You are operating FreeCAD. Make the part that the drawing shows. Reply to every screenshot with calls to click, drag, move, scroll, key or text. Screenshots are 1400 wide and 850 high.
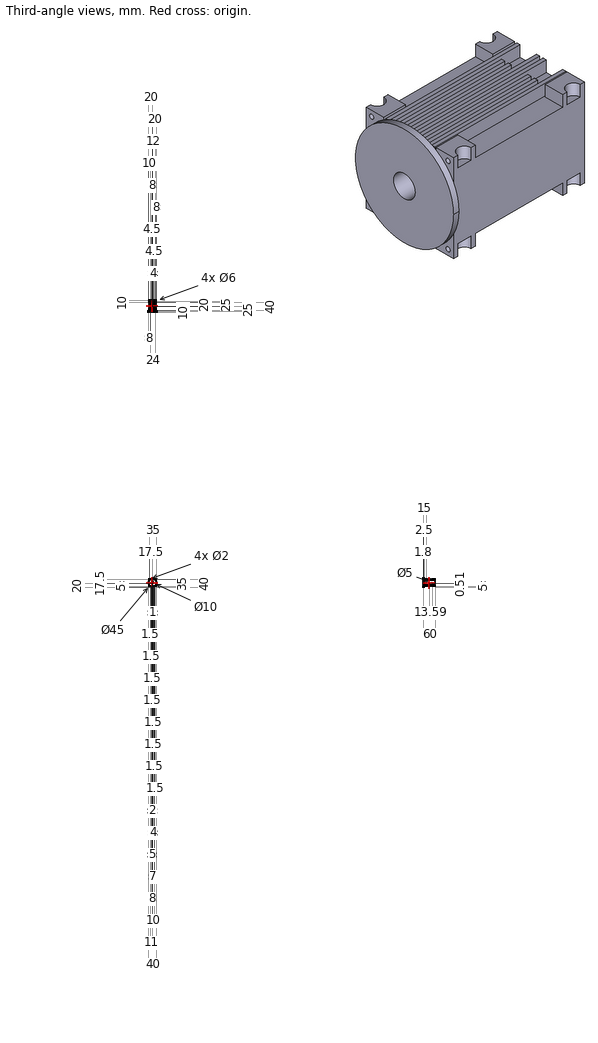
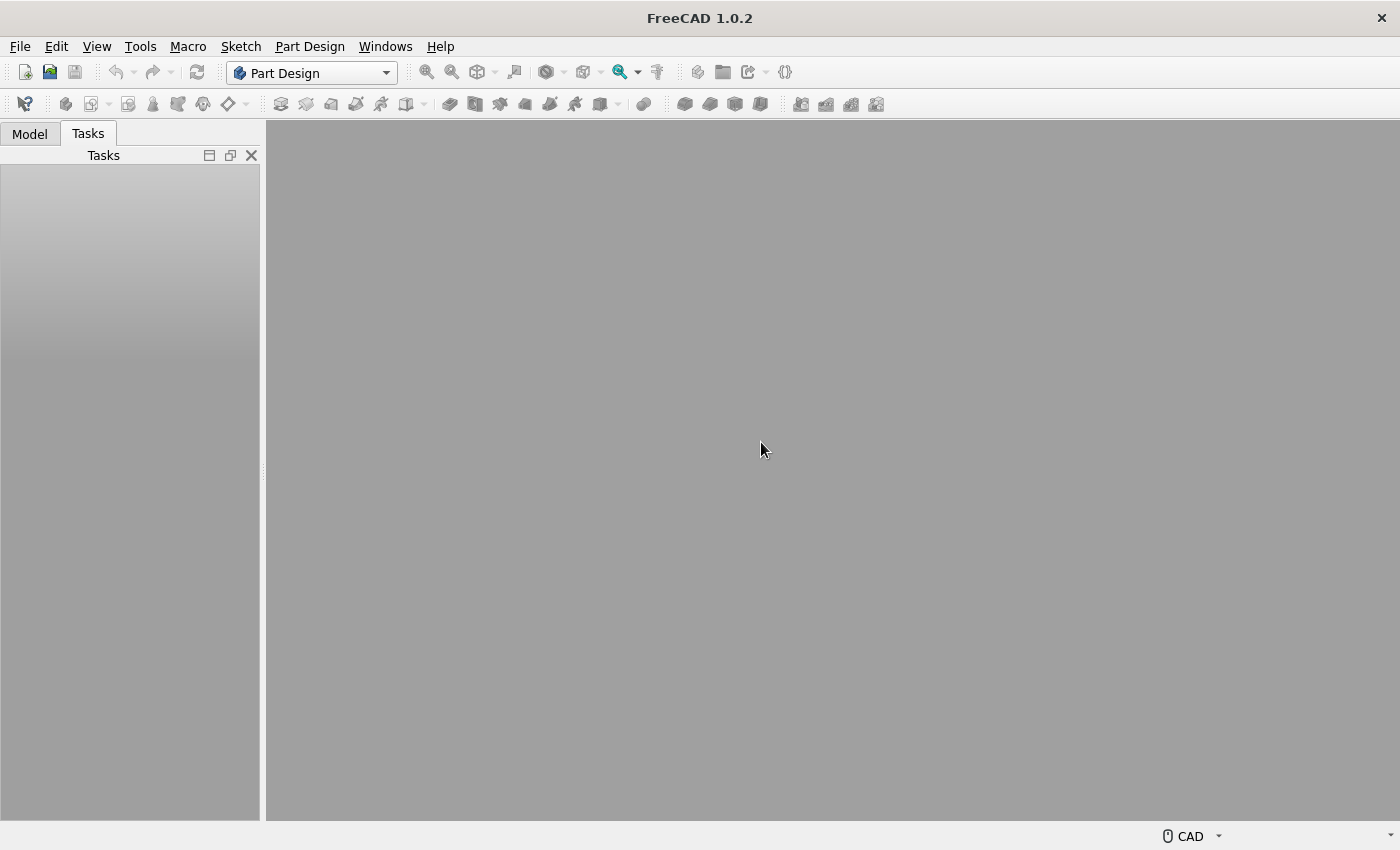
key(ctrl+n)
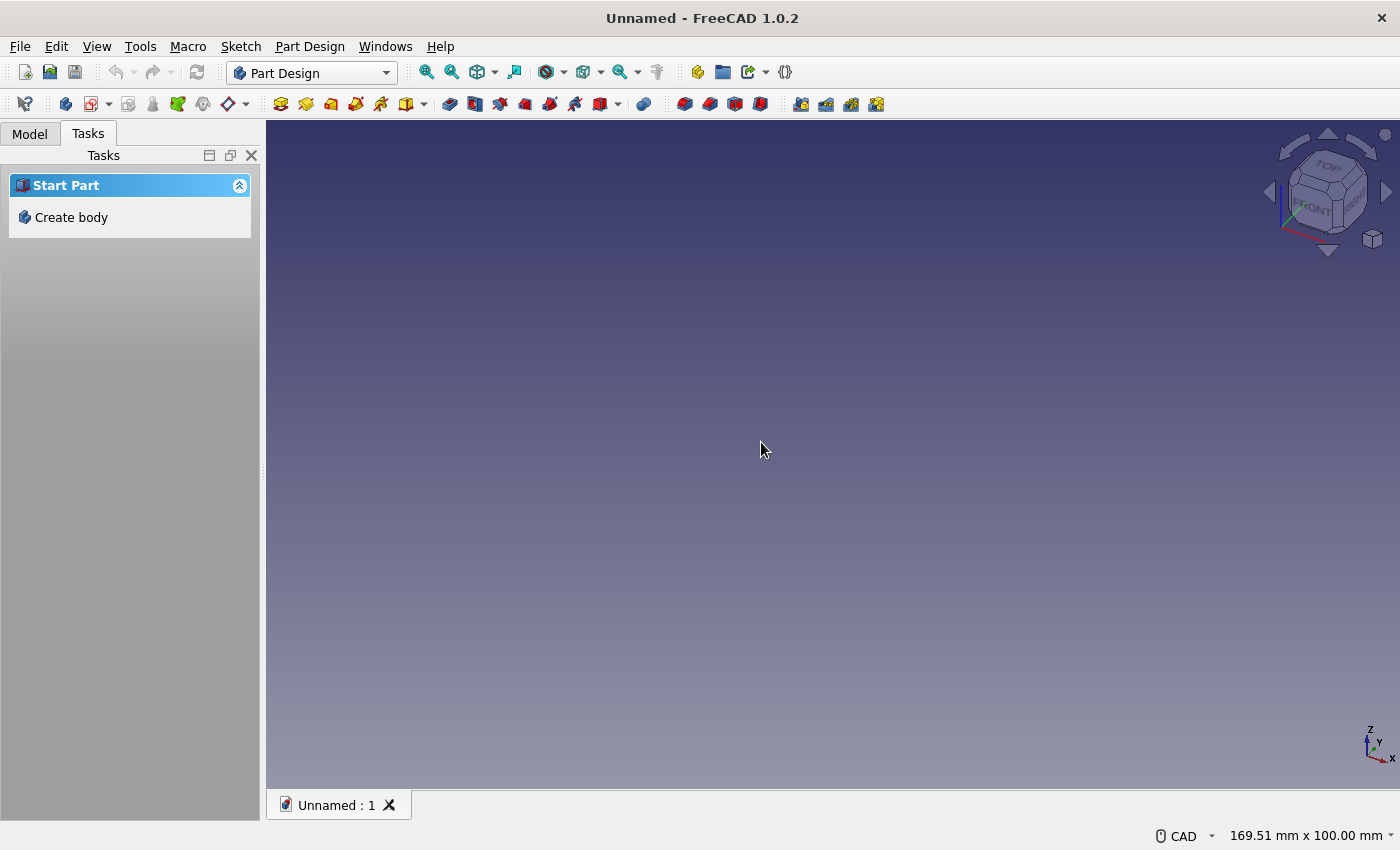
click(90, 104)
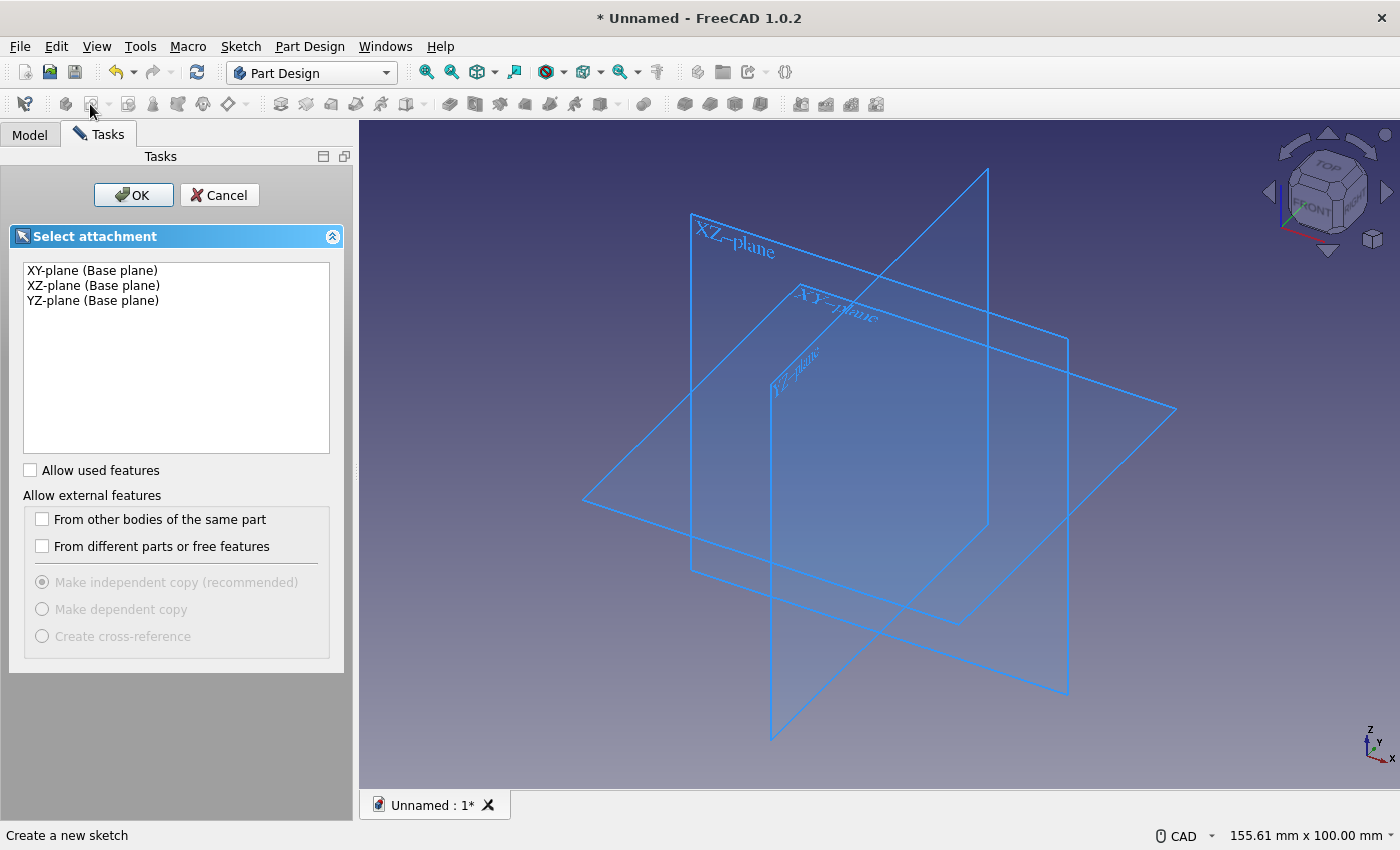
click(84, 286)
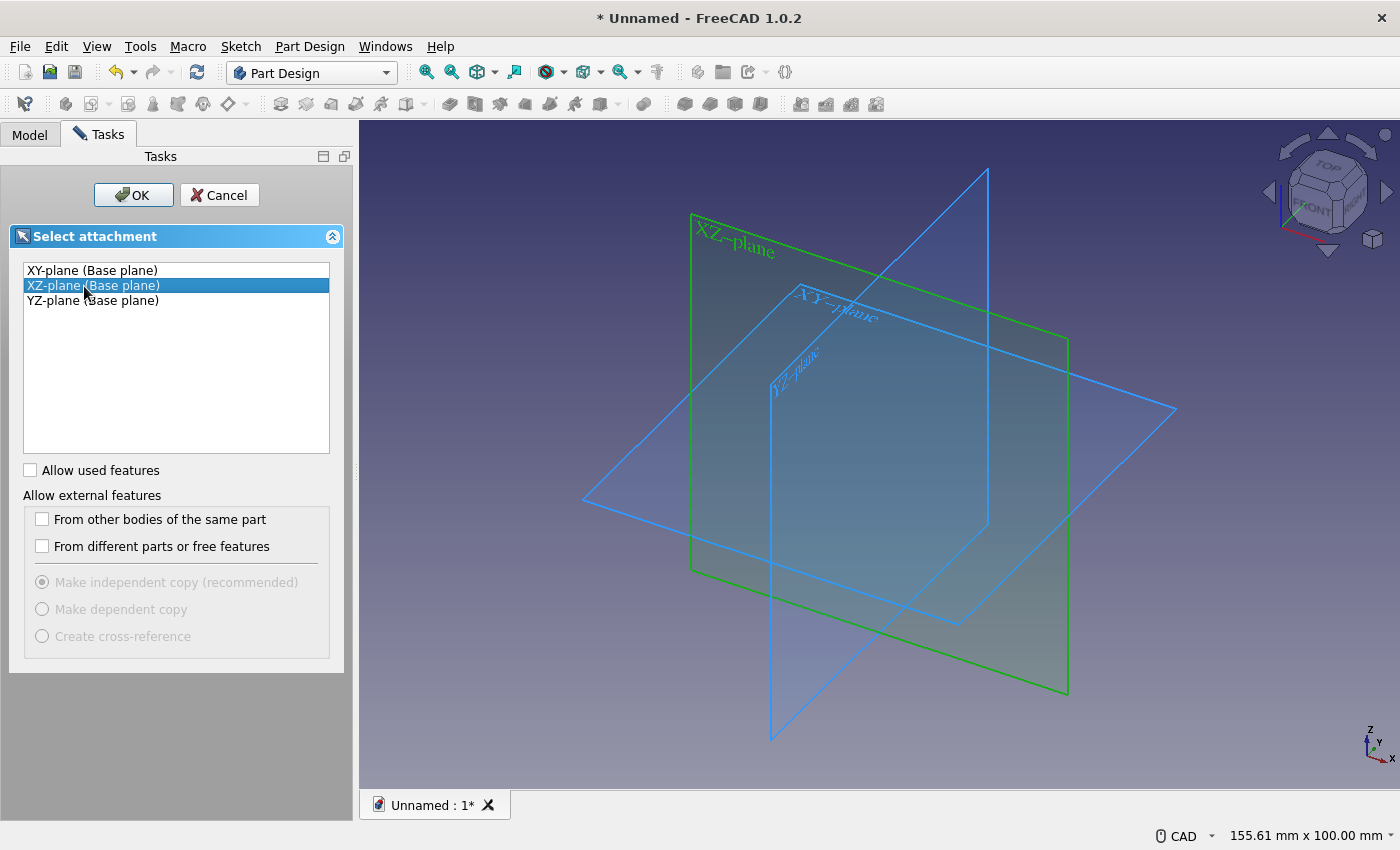
click(134, 195)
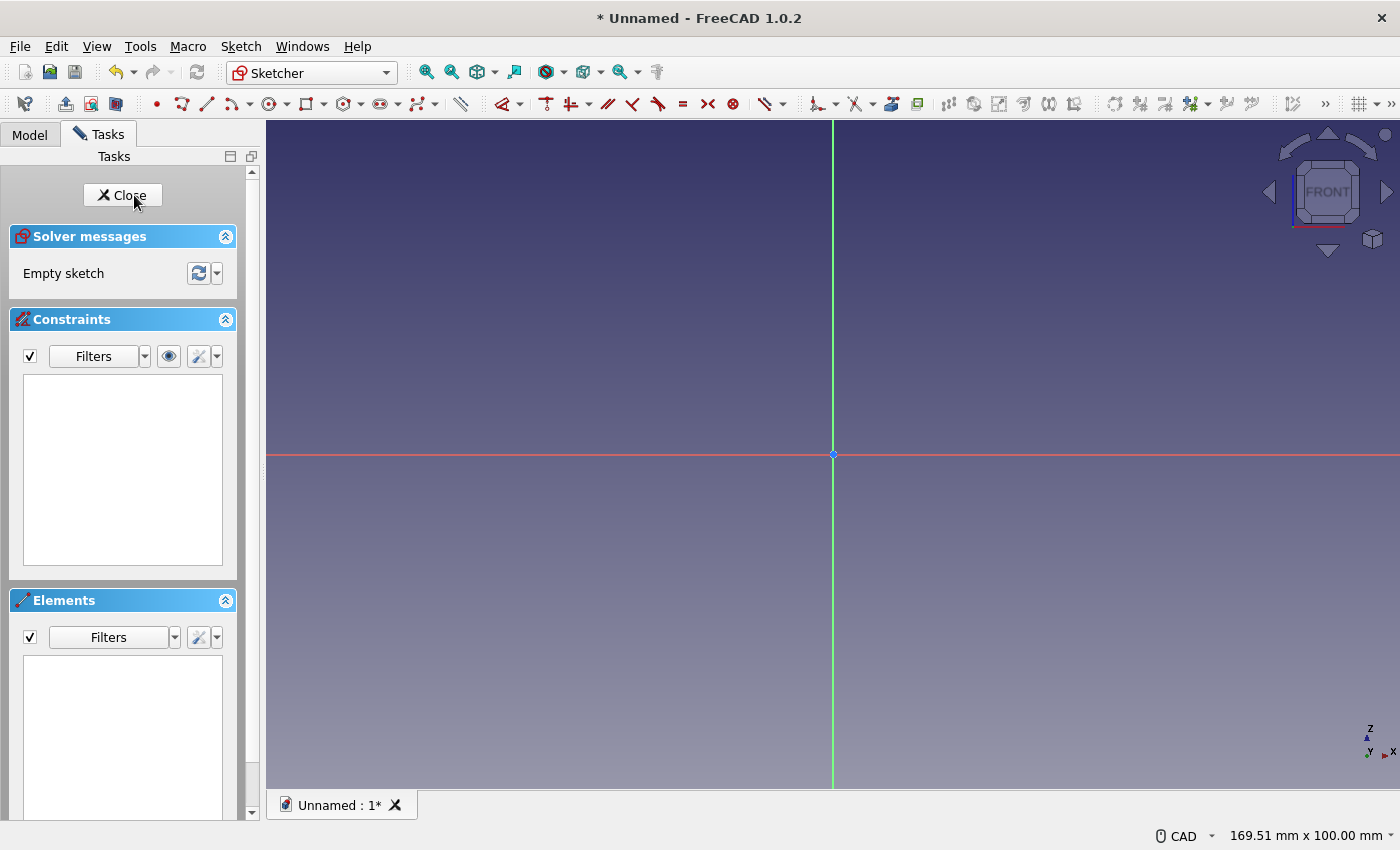
scroll(972, 455, up, 2)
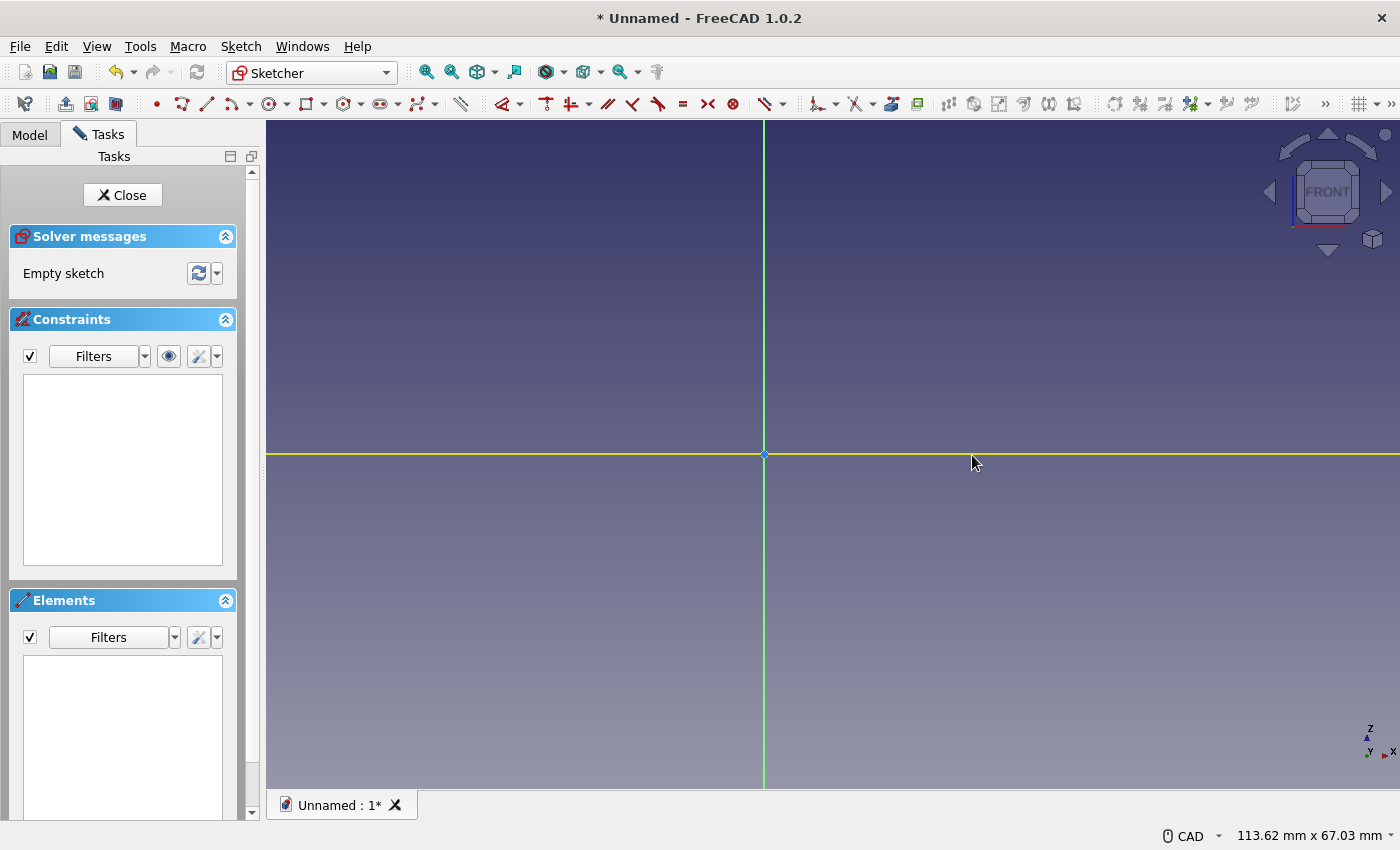
click(324, 104)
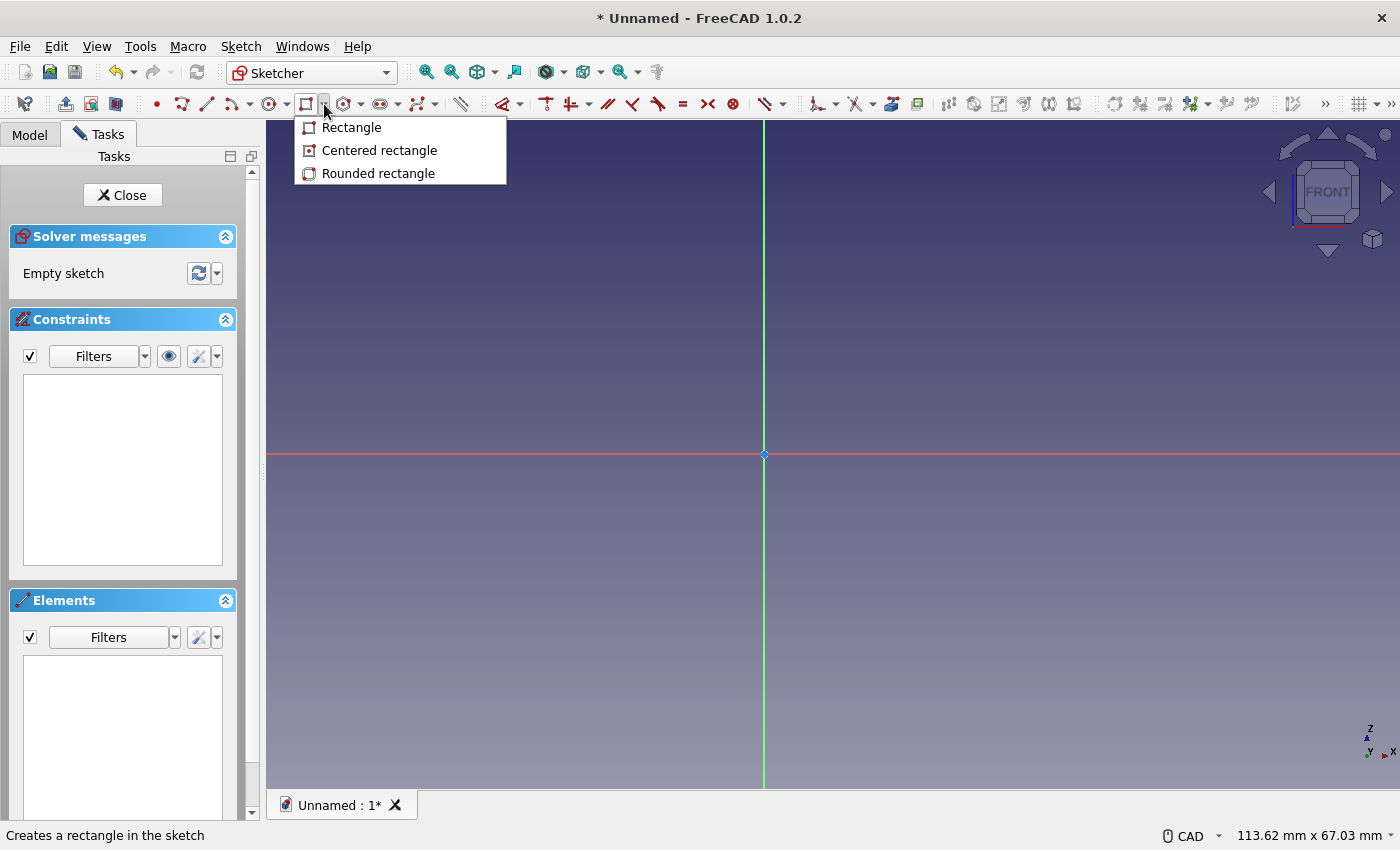
click(400, 150)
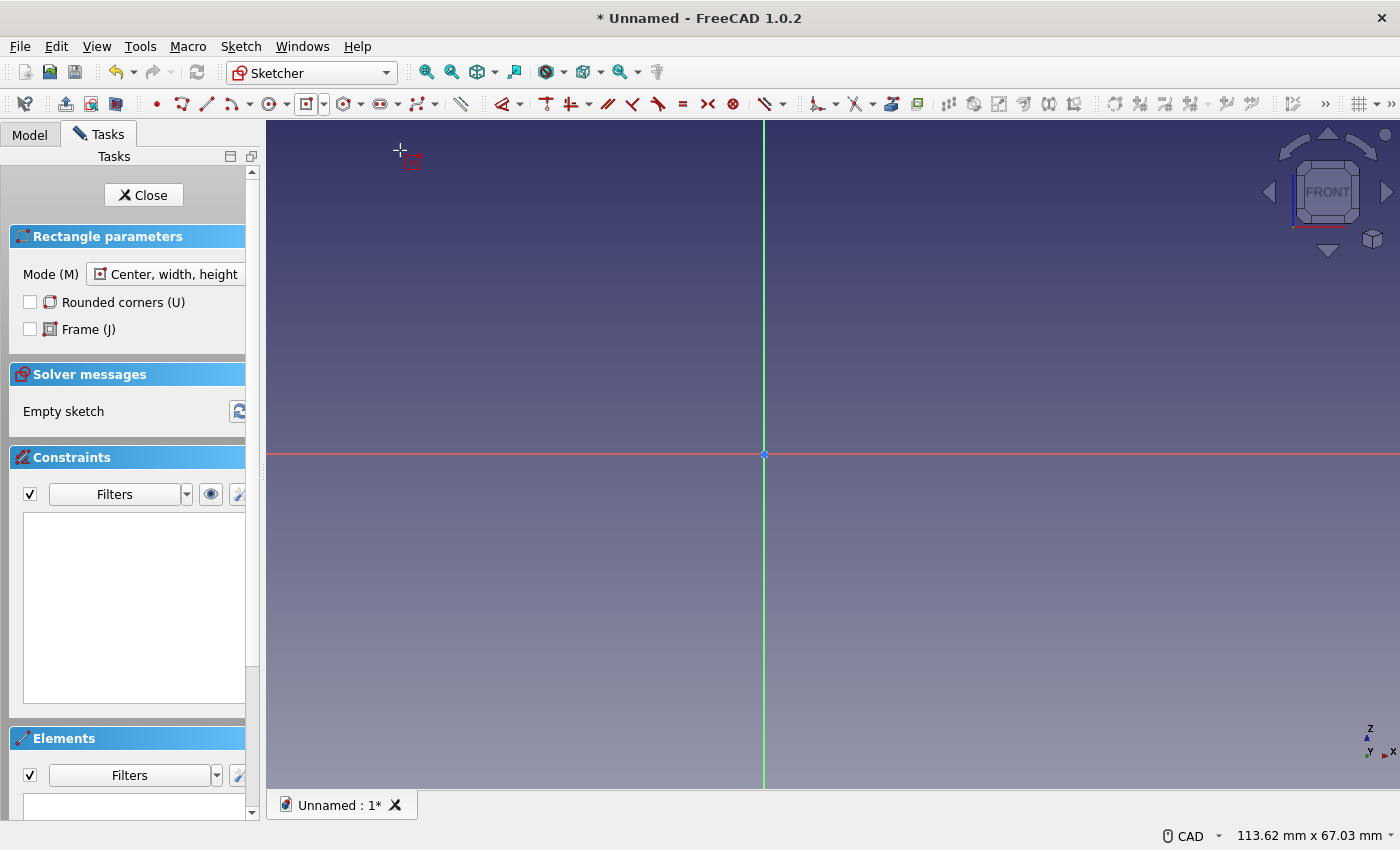
click(764, 454)
click(964, 254)
key(Escape)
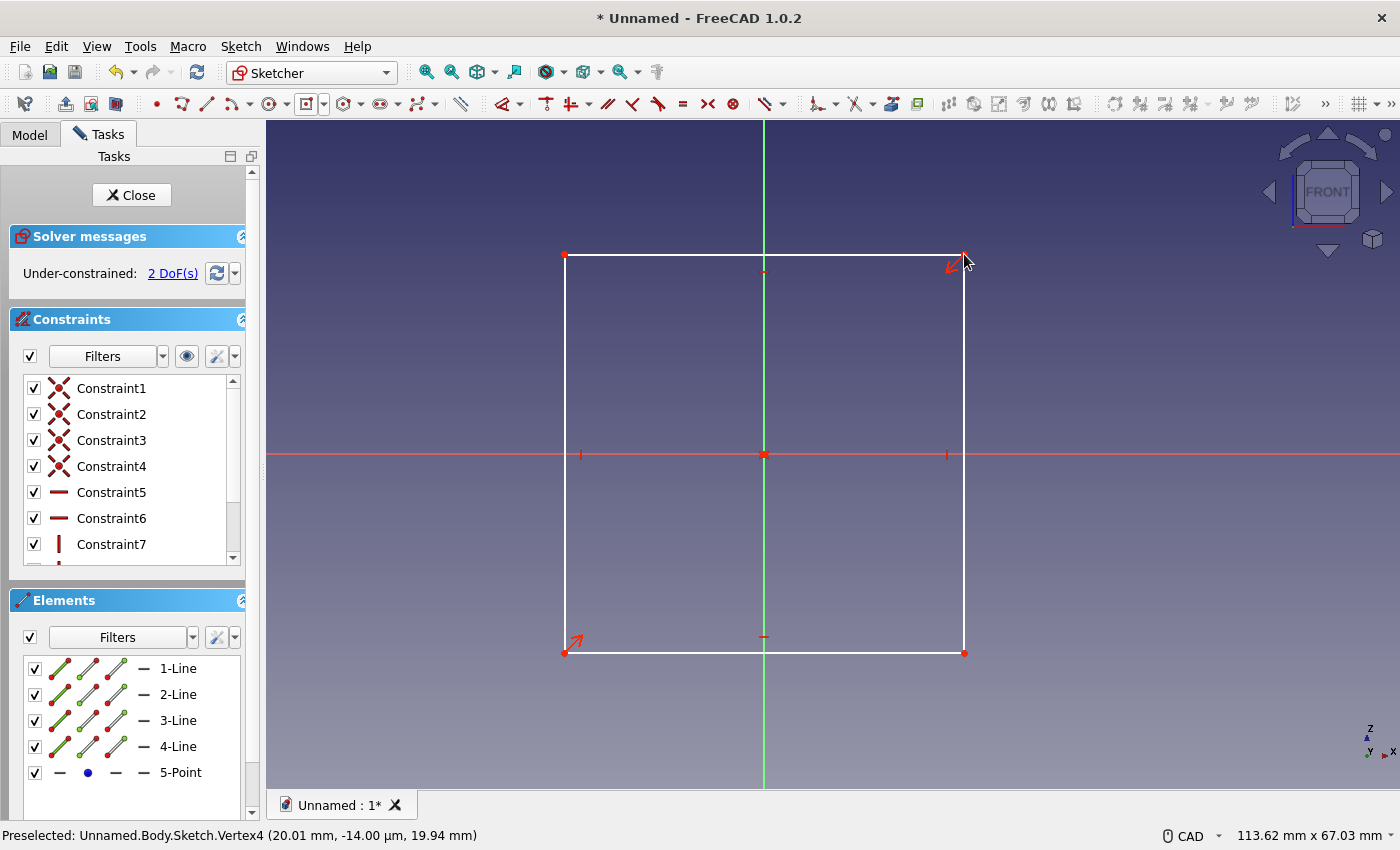
click(502, 104)